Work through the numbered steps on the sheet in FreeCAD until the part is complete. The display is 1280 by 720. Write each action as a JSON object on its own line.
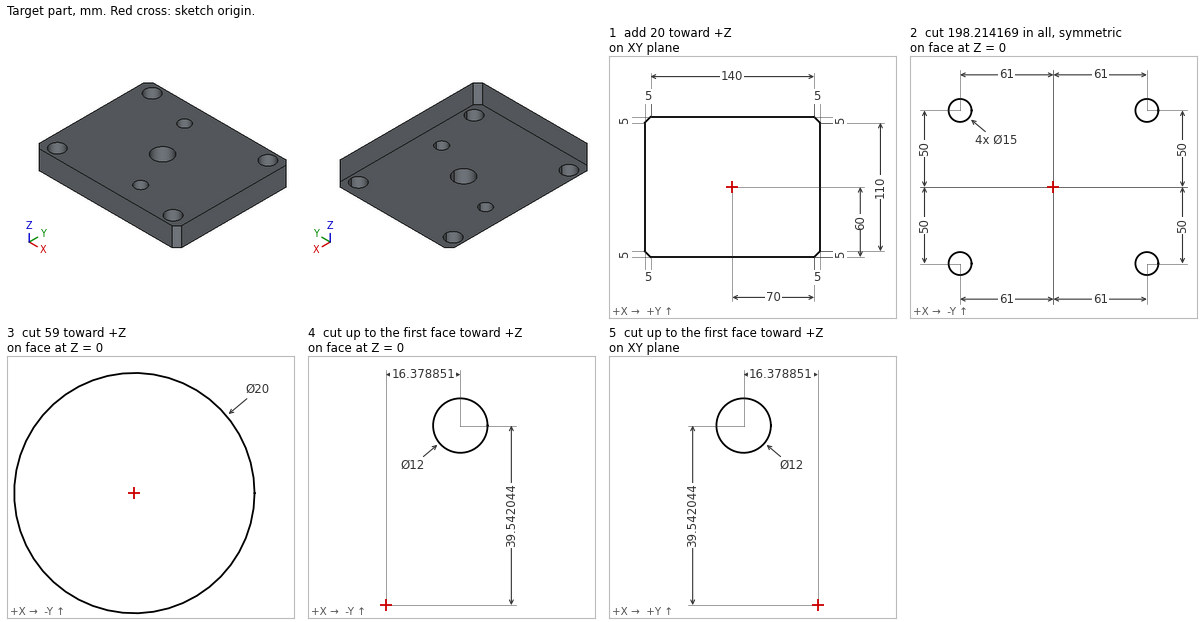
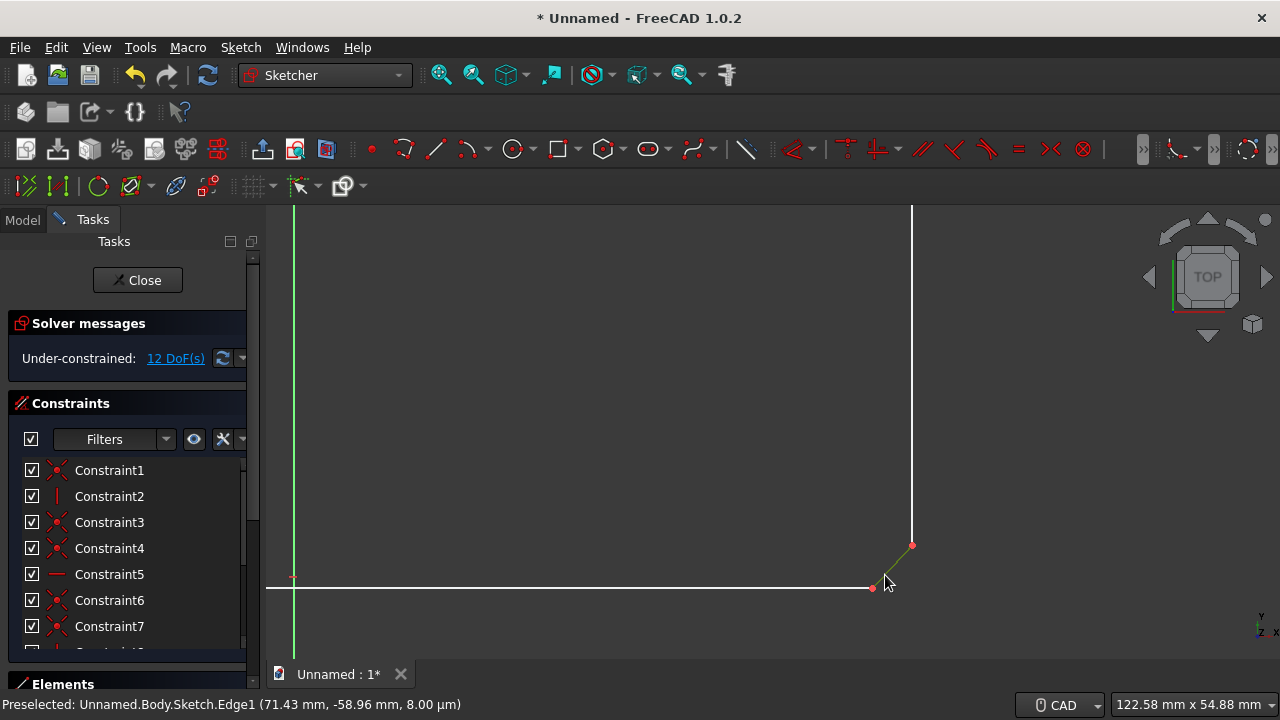
{"action": "key", "text": "l"}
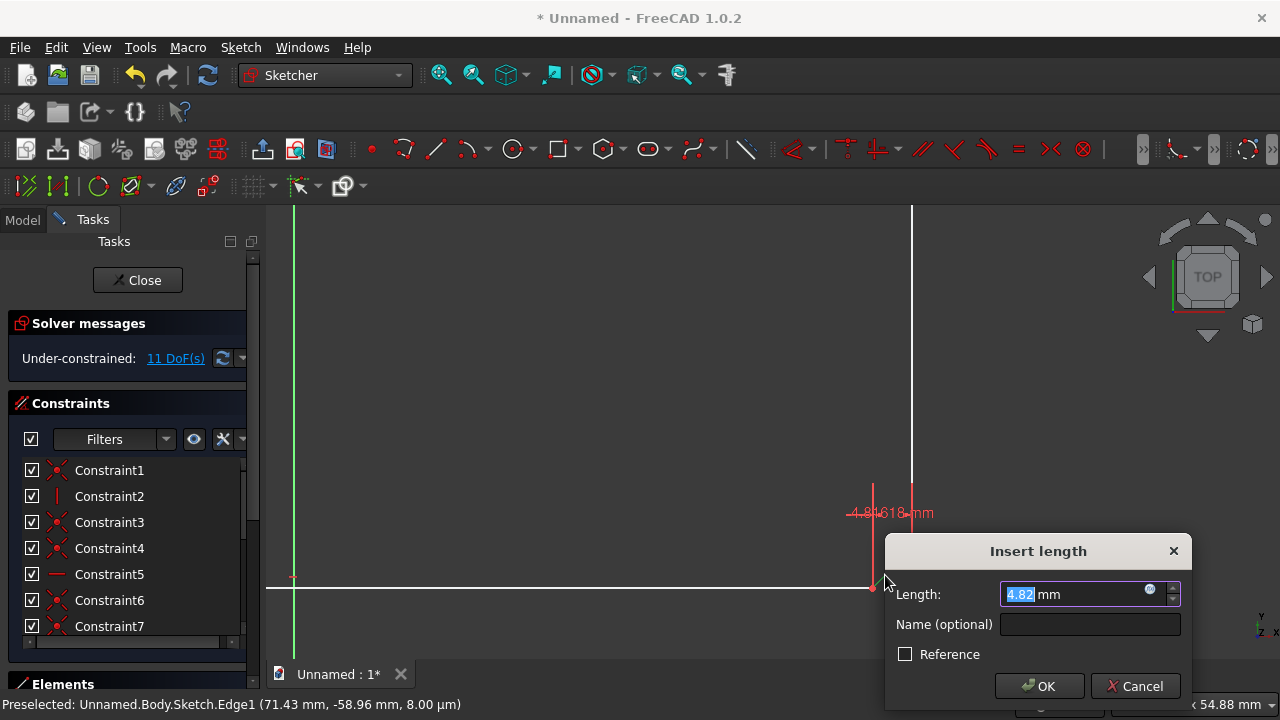
{"action": "type", "text": "5"}
{"action": "key", "text": "Return"}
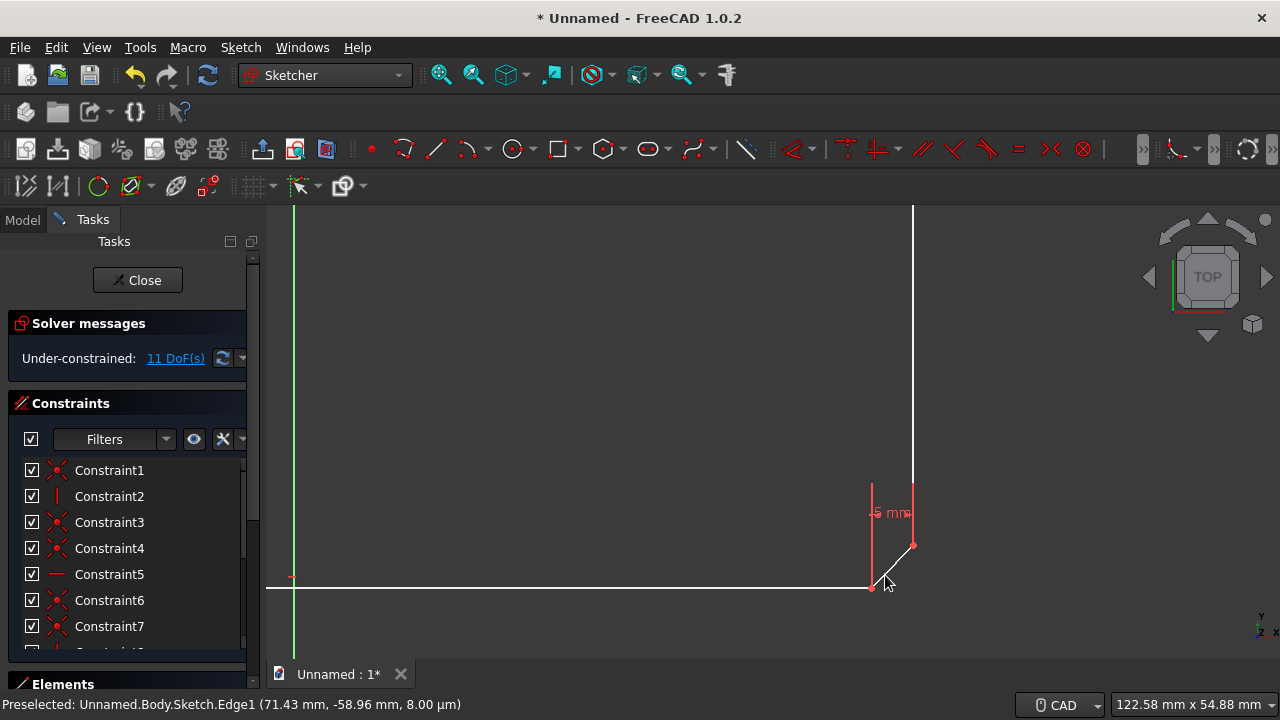
{"action": "left_click", "coordinate": [884, 575]}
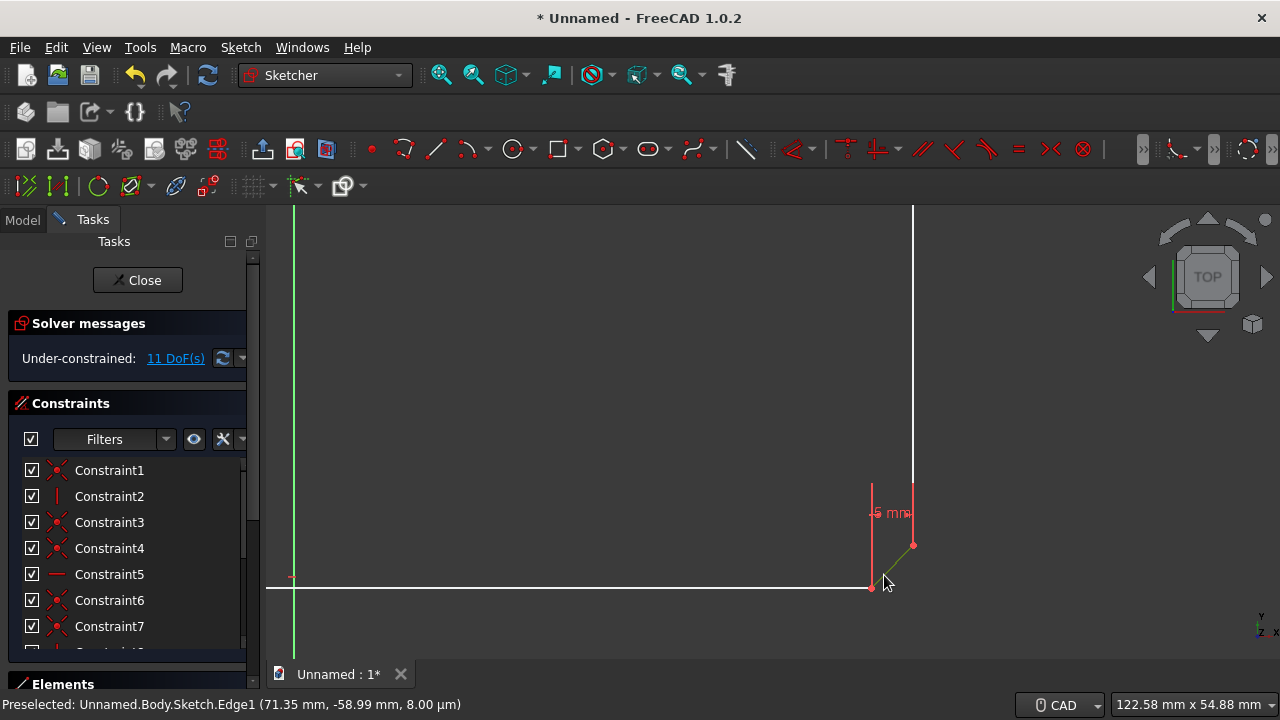
{"action": "key", "text": "i"}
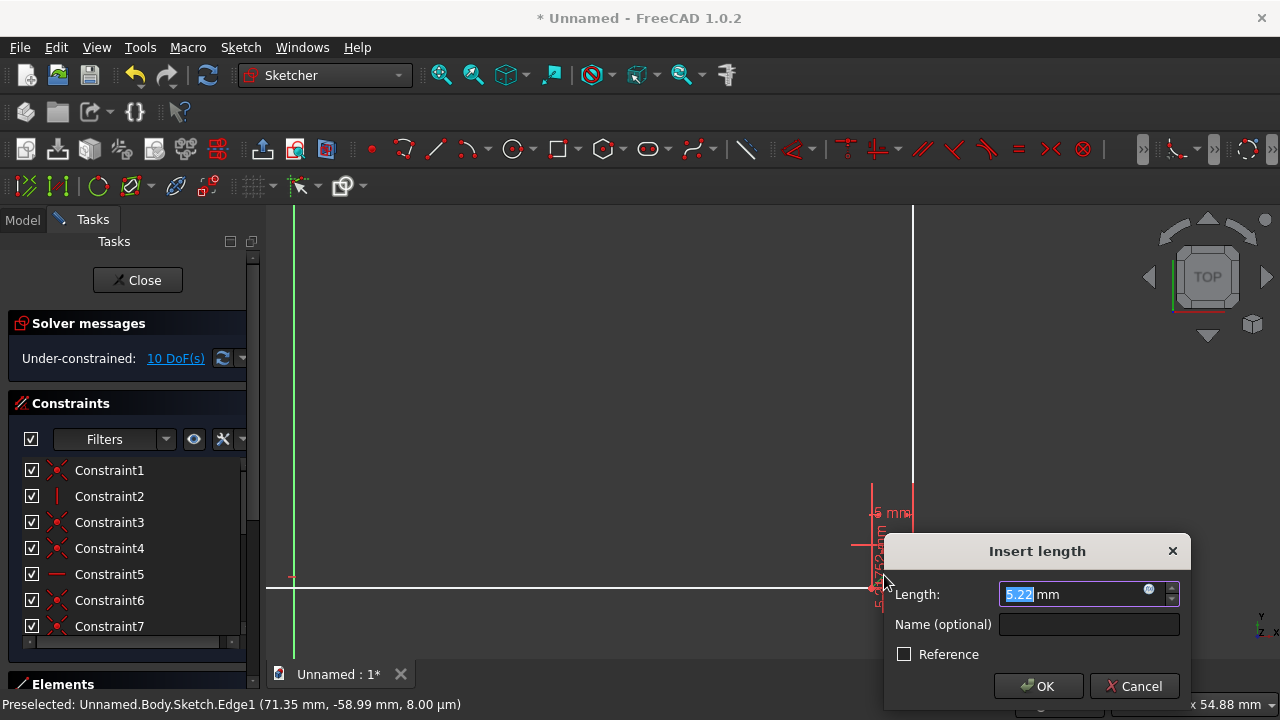
{"action": "type", "text": "5"}
{"action": "key", "text": "Return"}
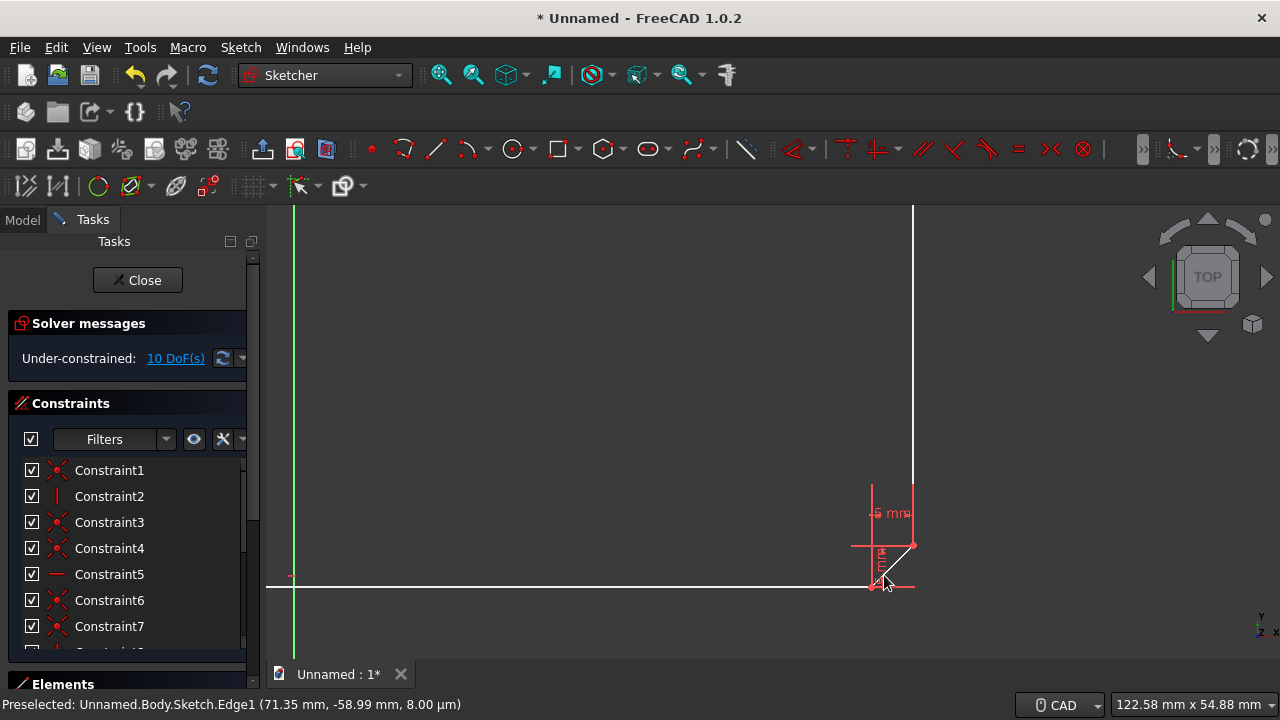
{"action": "scroll", "coordinate": [882, 580], "scroll_direction": "down", "scroll_amount": 6}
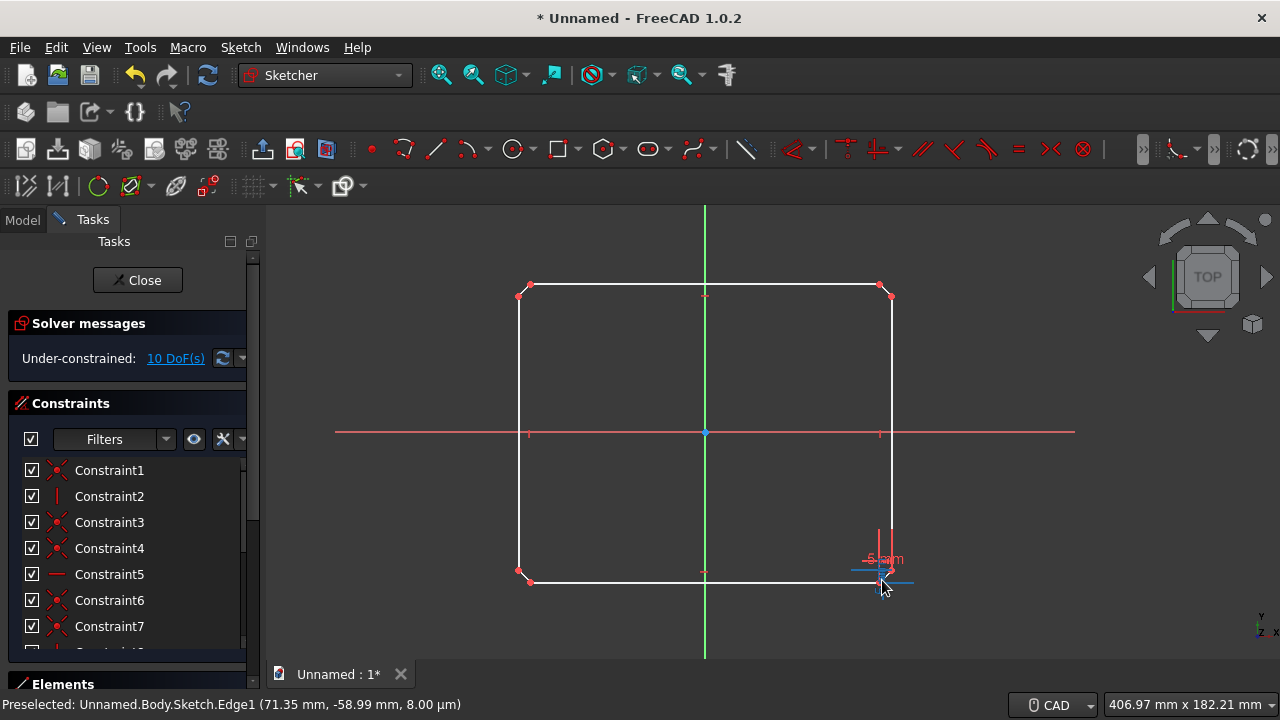
{"action": "scroll", "coordinate": [888, 292], "scroll_direction": "up", "scroll_amount": 6}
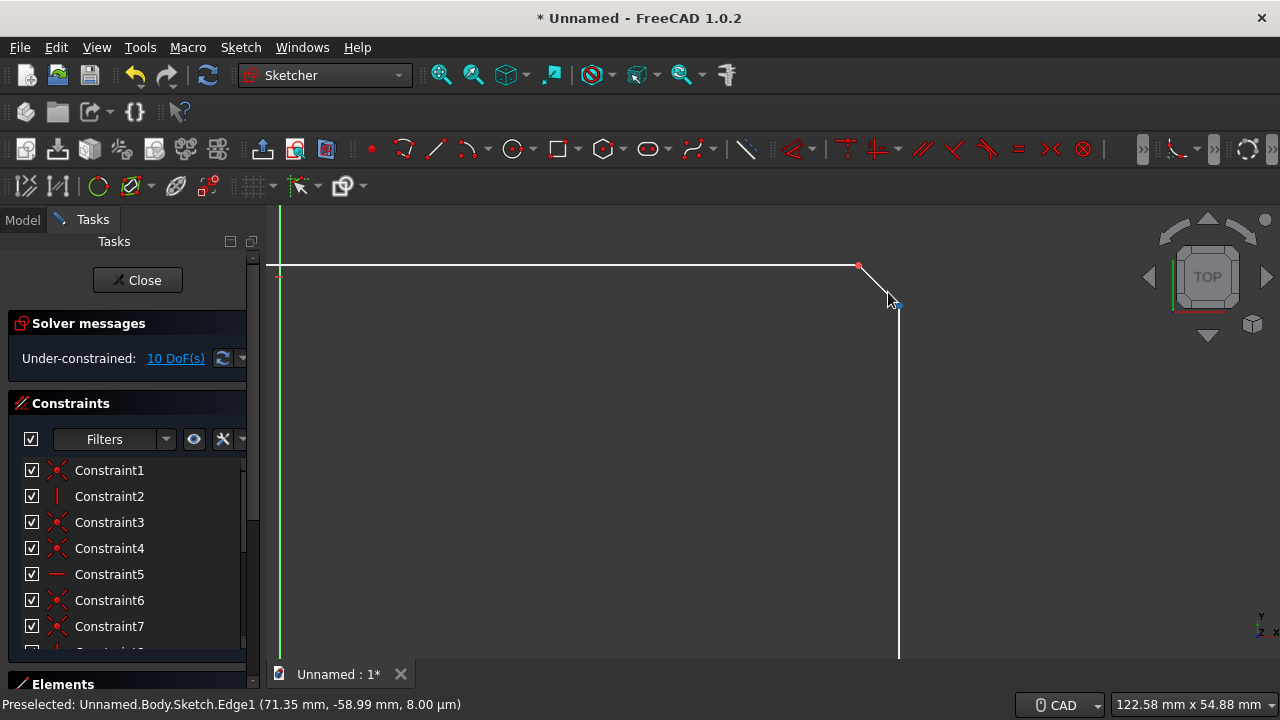
{"action": "left_click", "coordinate": [887, 293]}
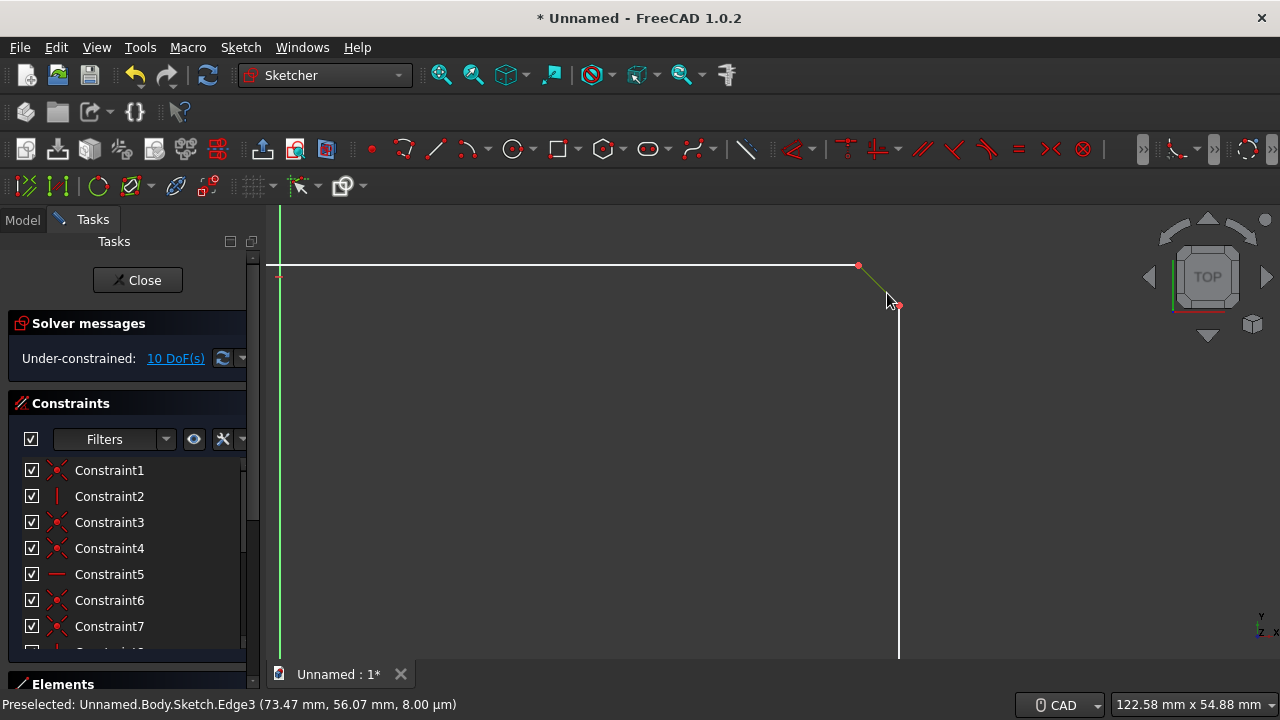
{"action": "key", "text": "l"}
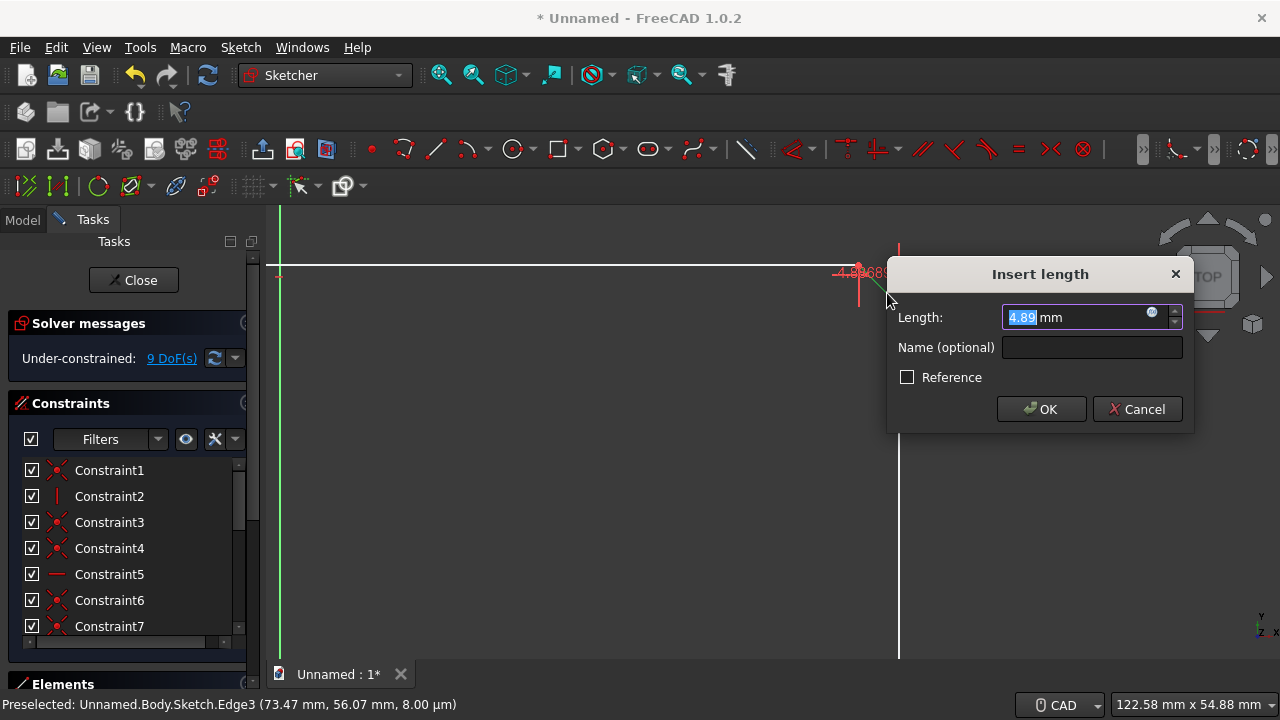
{"action": "type", "text": "5"}
{"action": "key", "text": "Return"}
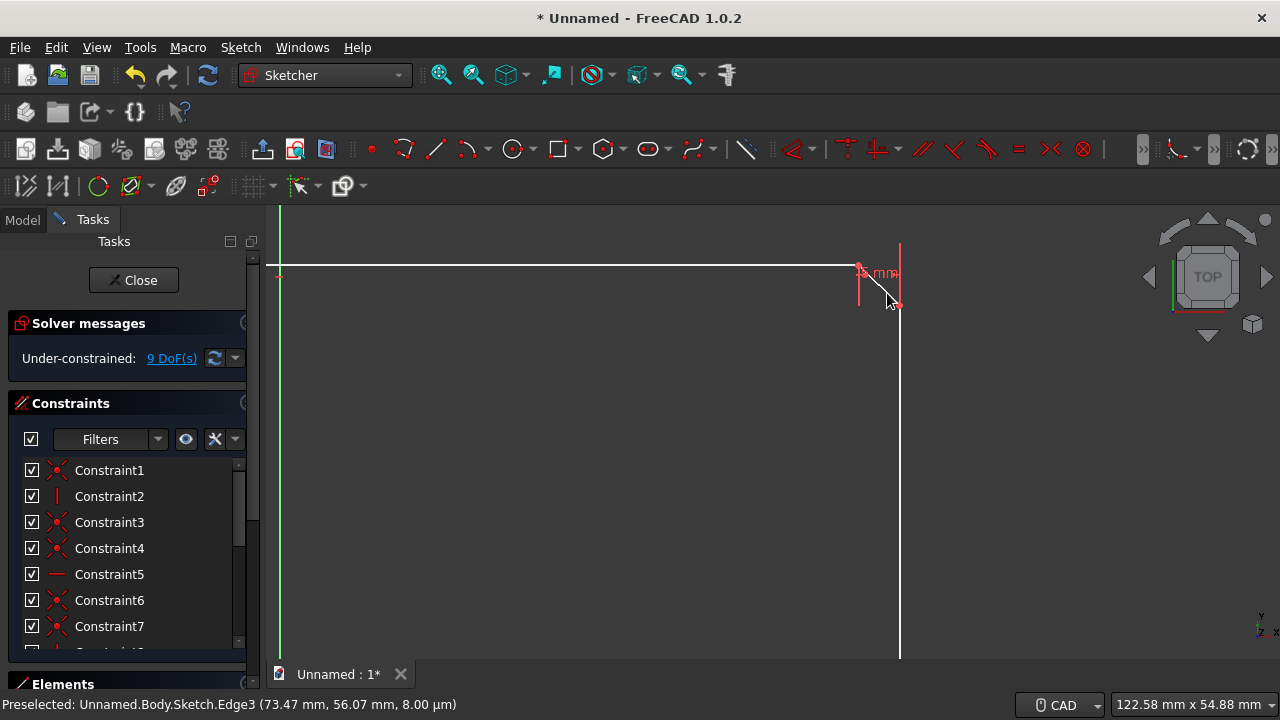
{"action": "left_click", "coordinate": [887, 293]}